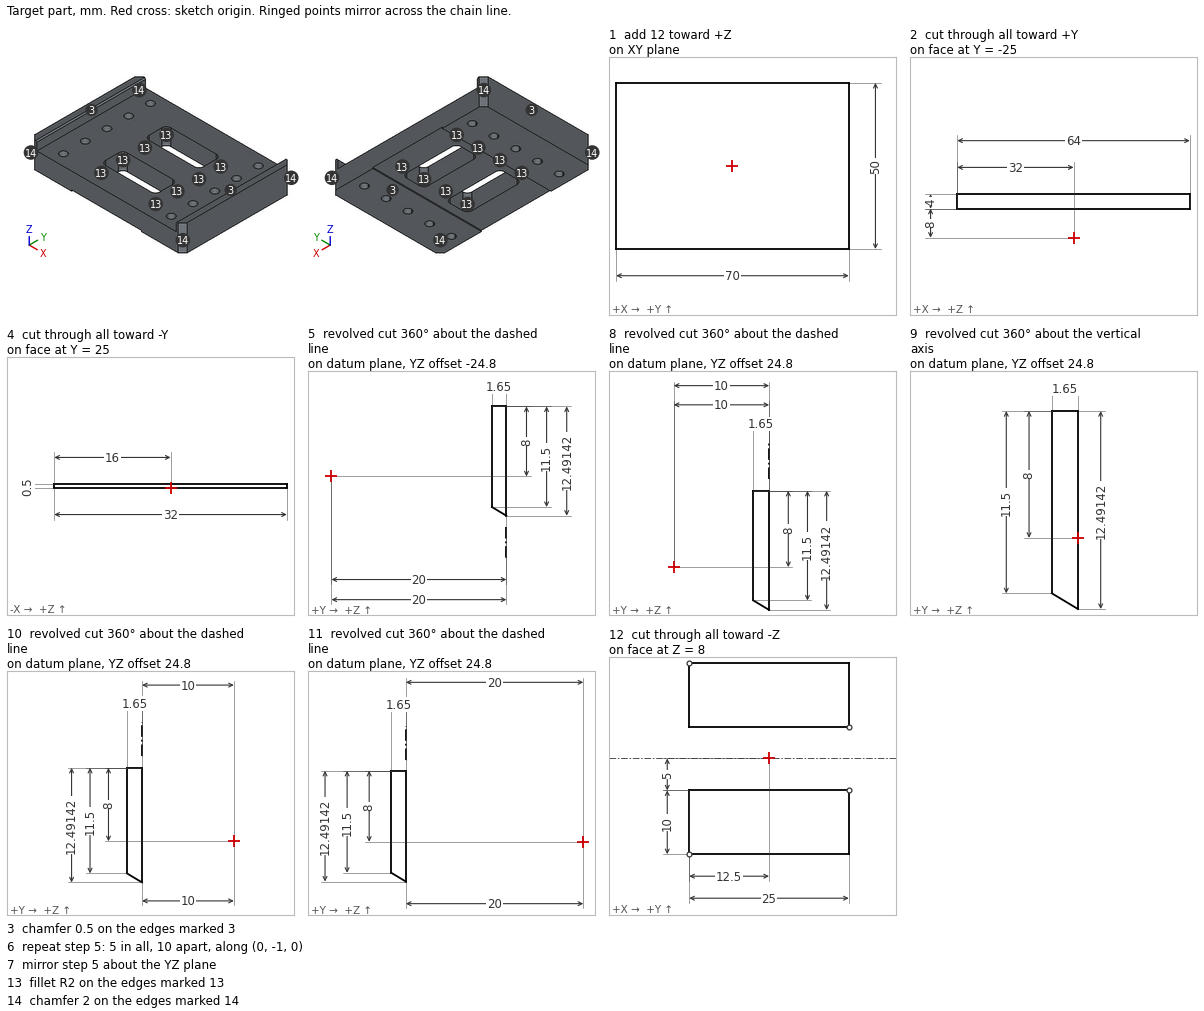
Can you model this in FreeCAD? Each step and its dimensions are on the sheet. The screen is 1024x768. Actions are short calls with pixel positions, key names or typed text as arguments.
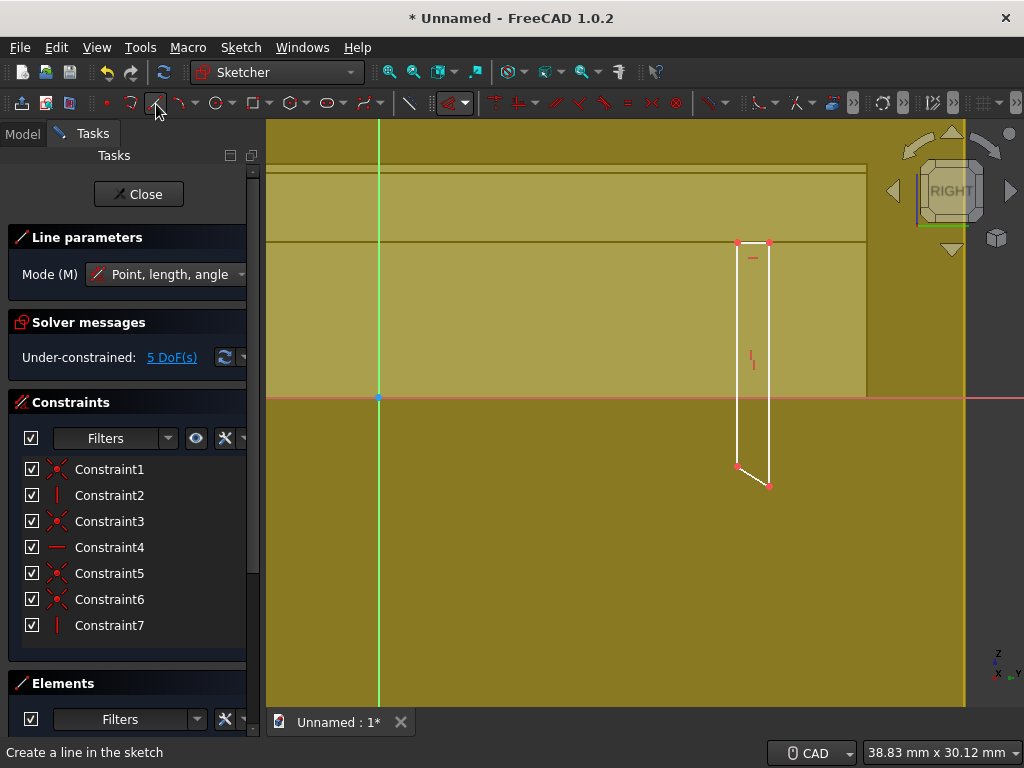
click(769, 510)
click(769, 583)
key(Escape)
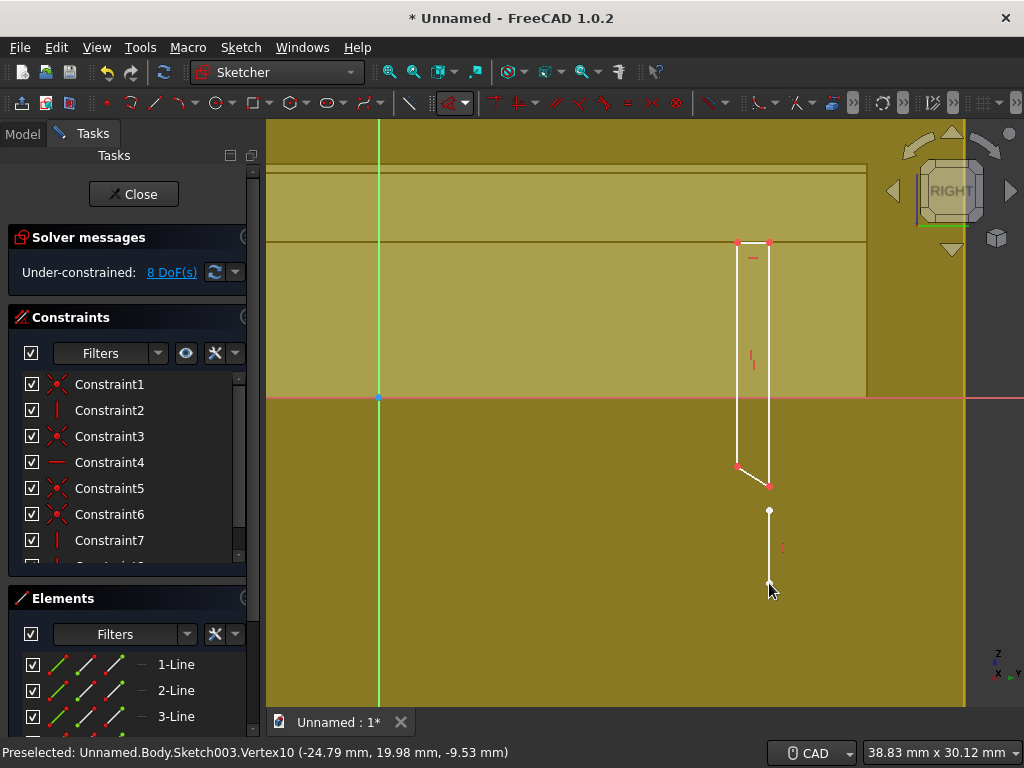
click(769, 533)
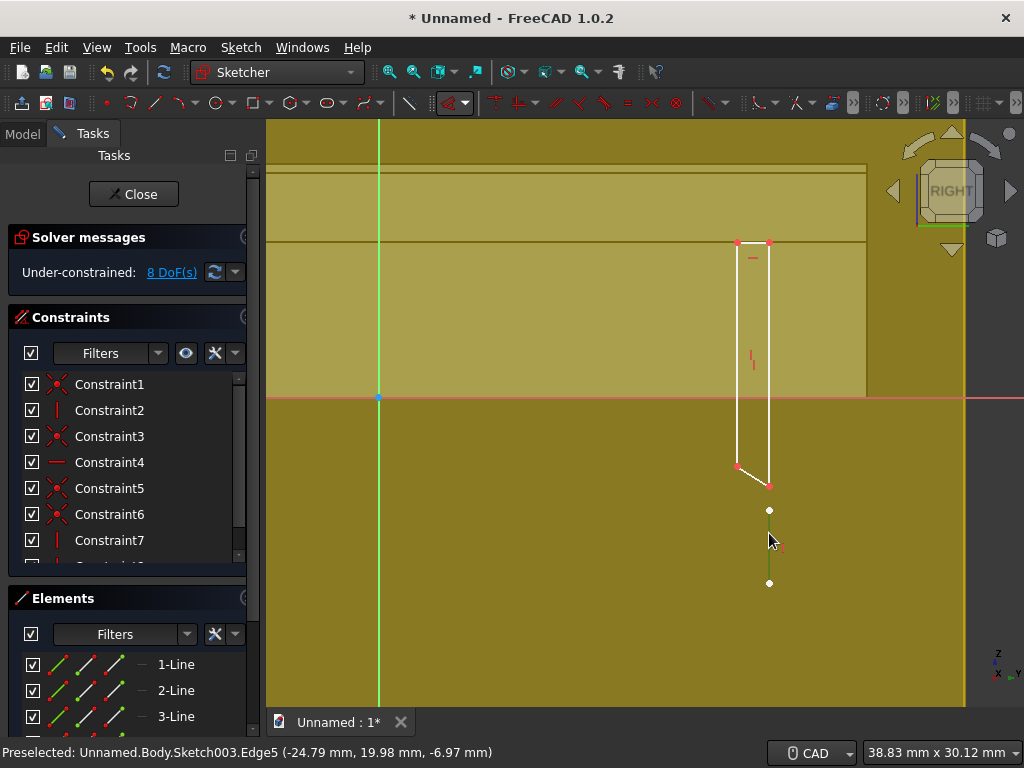
click(410, 104)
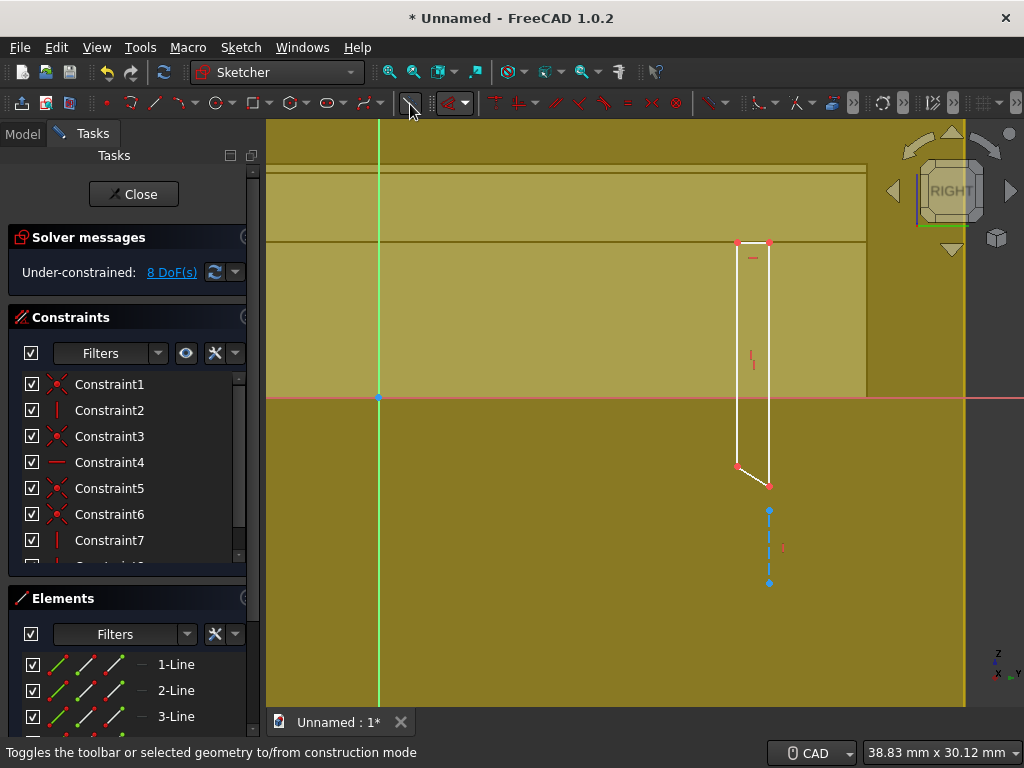
click(769, 243)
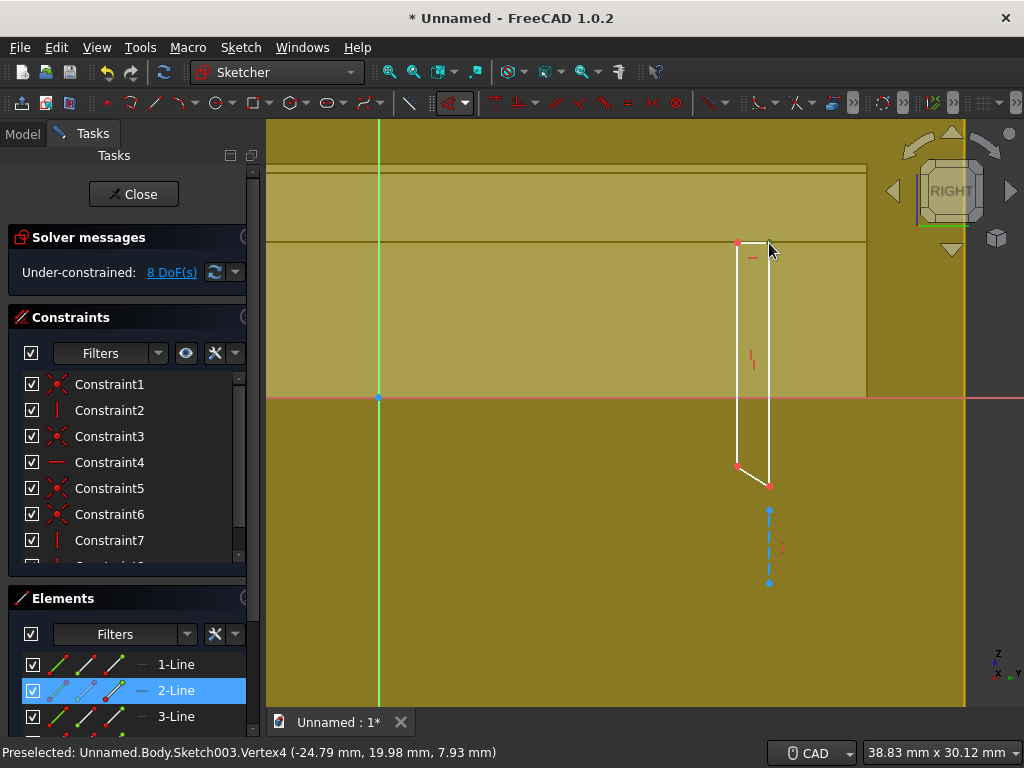
key(i)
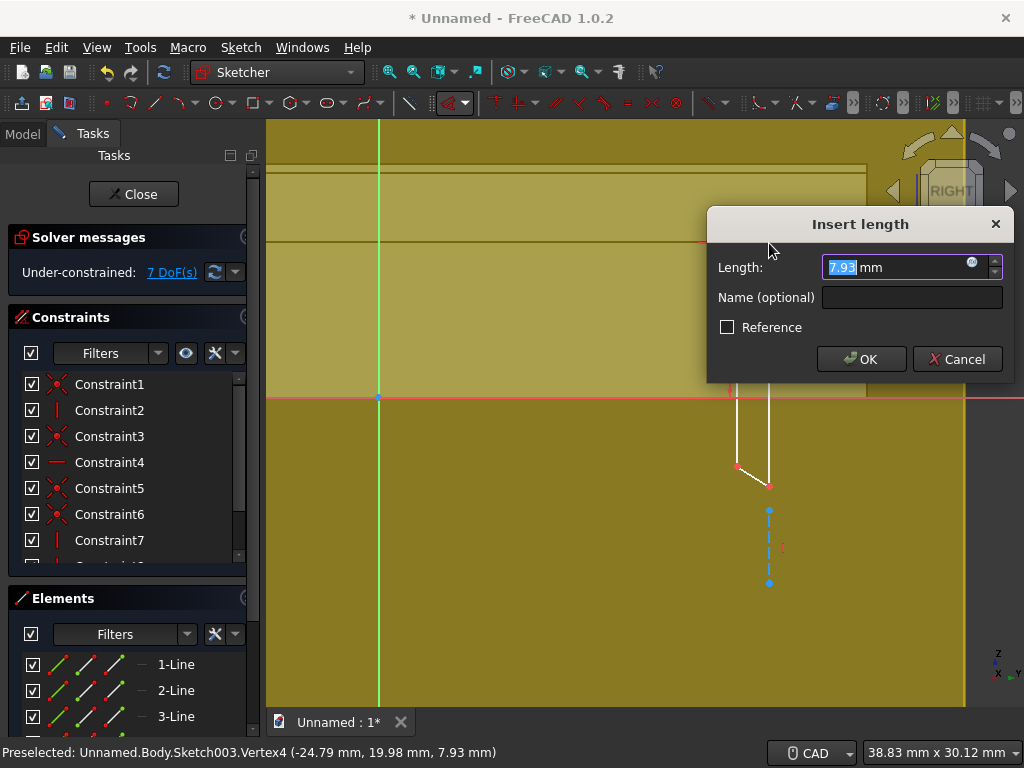
text(8)
key(Return)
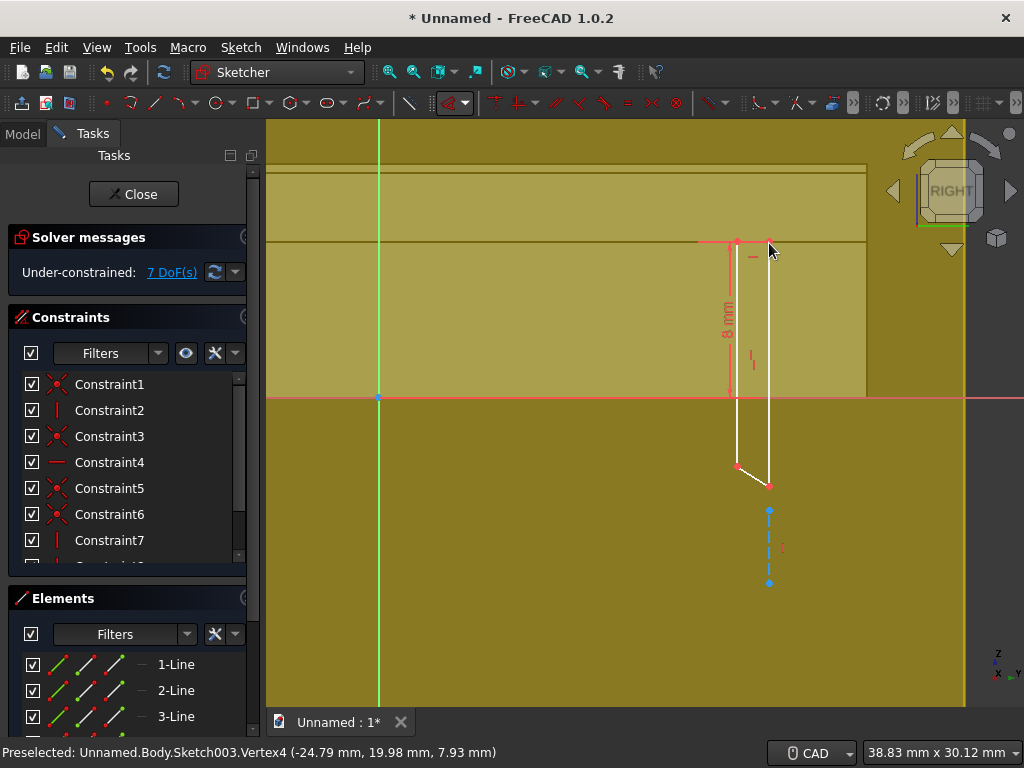
click(769, 487)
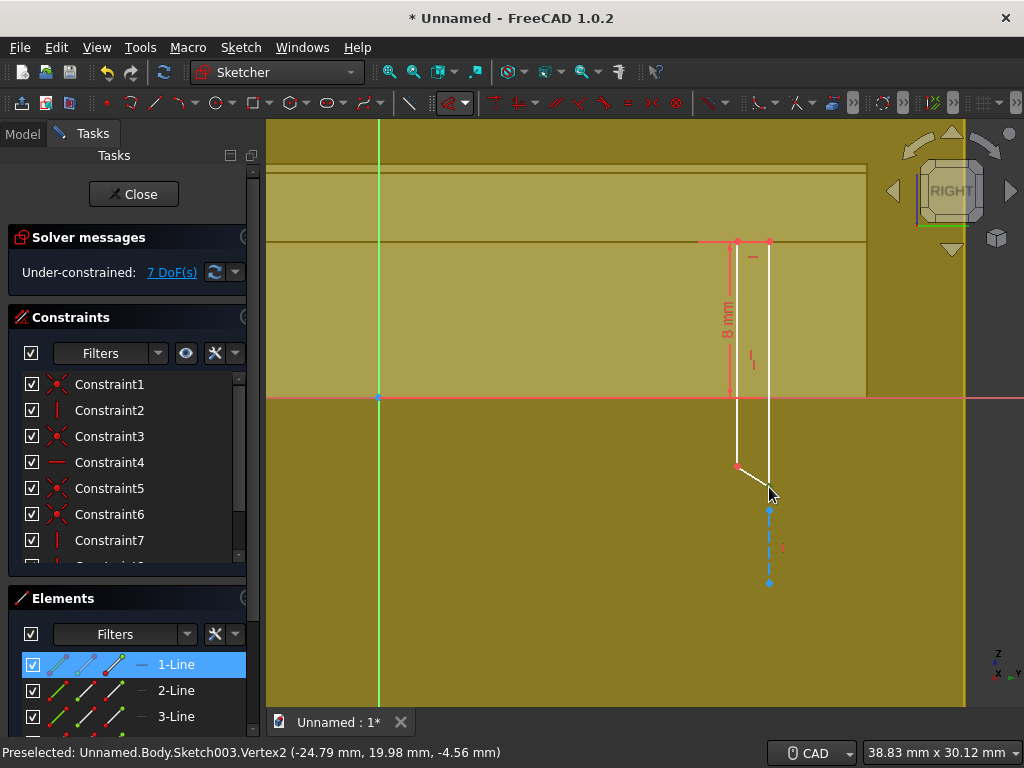
key(l)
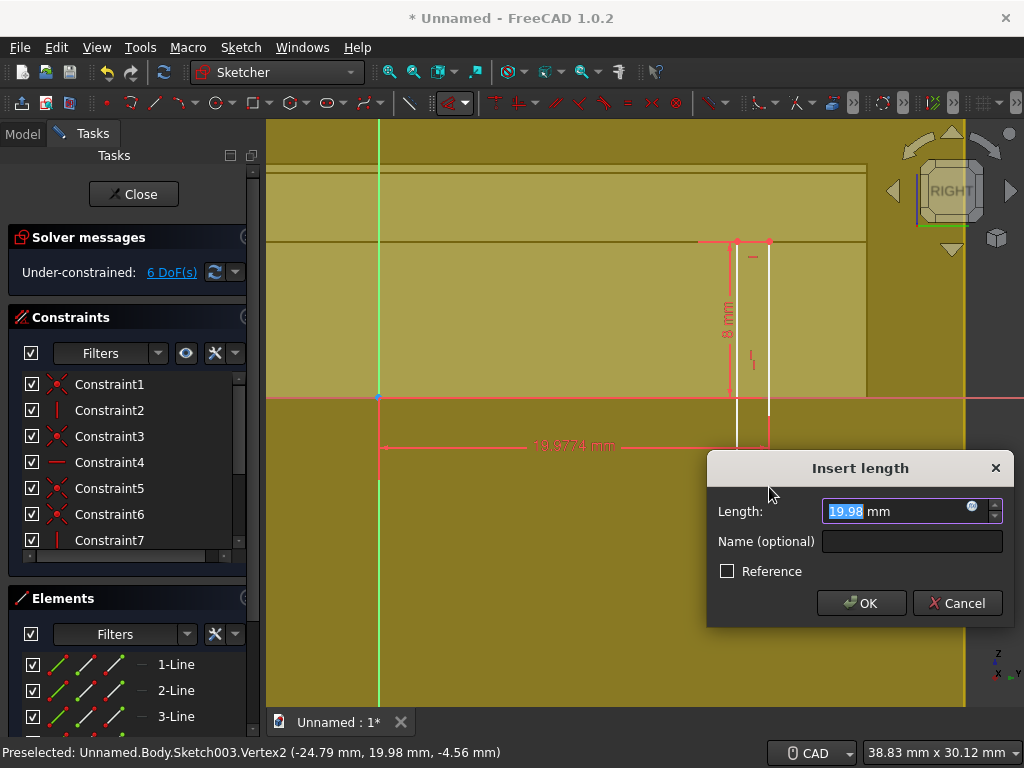
text(20)
key(Return)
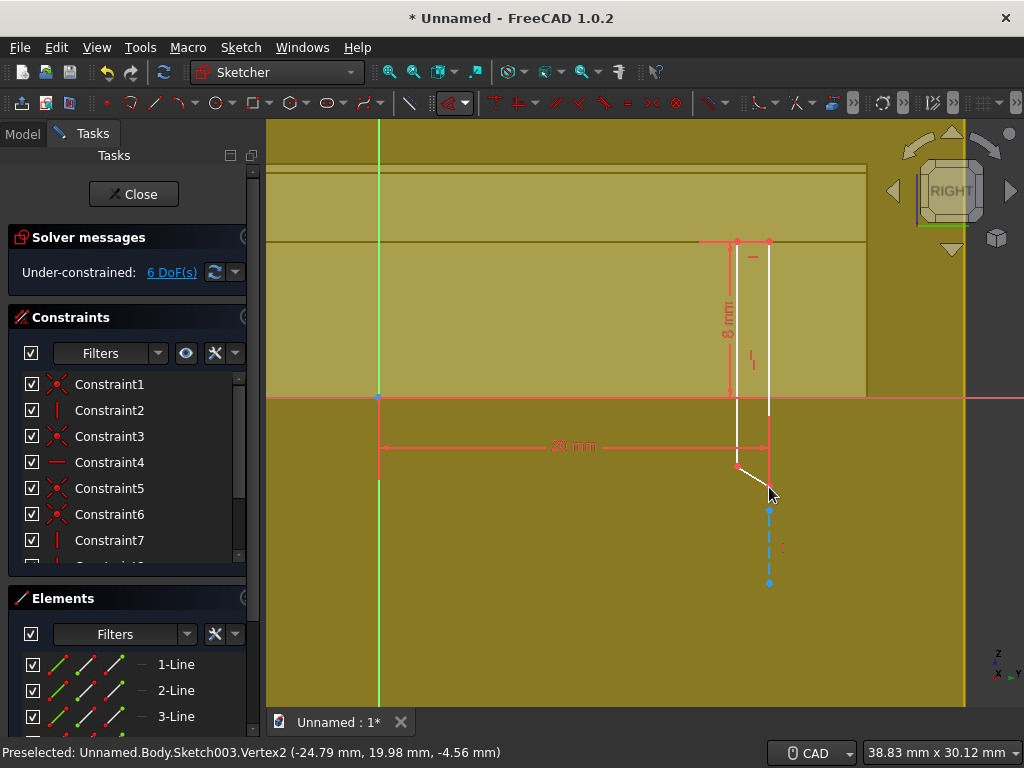
click(769, 511)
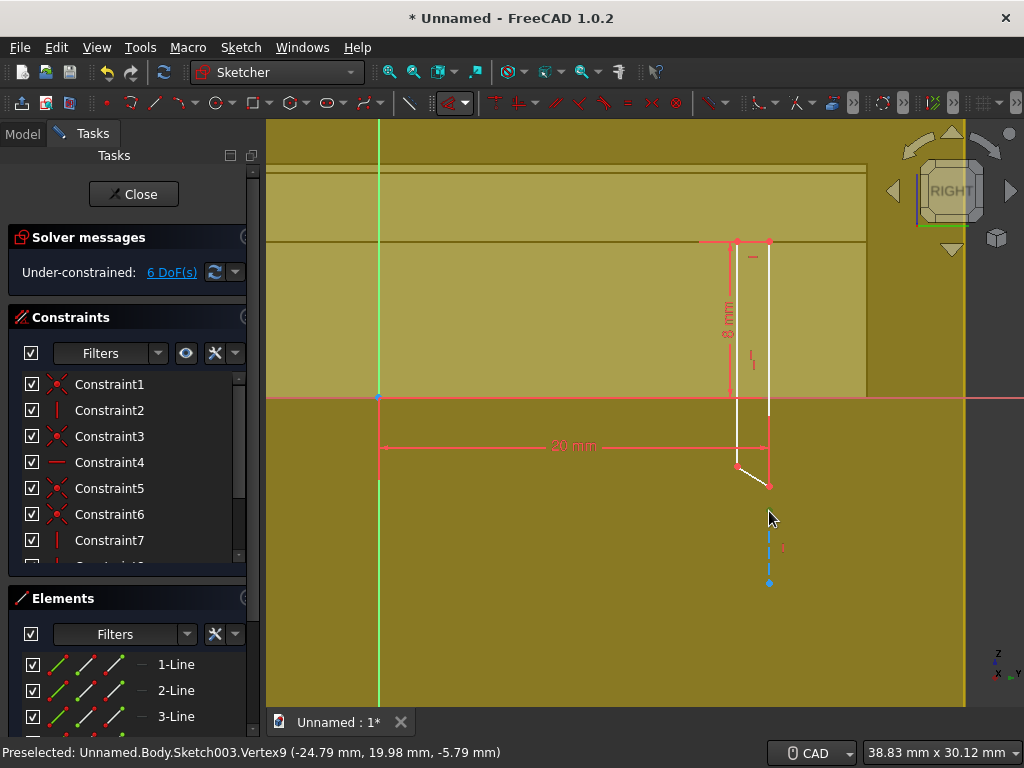
key(l)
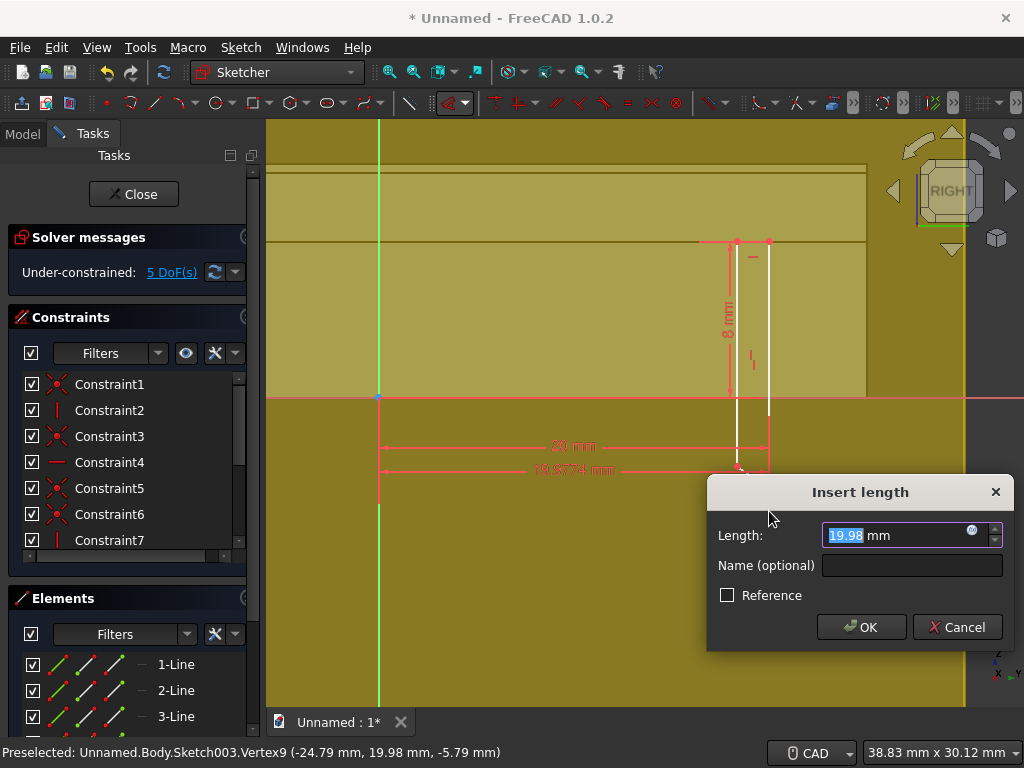
text(20)
key(Return)